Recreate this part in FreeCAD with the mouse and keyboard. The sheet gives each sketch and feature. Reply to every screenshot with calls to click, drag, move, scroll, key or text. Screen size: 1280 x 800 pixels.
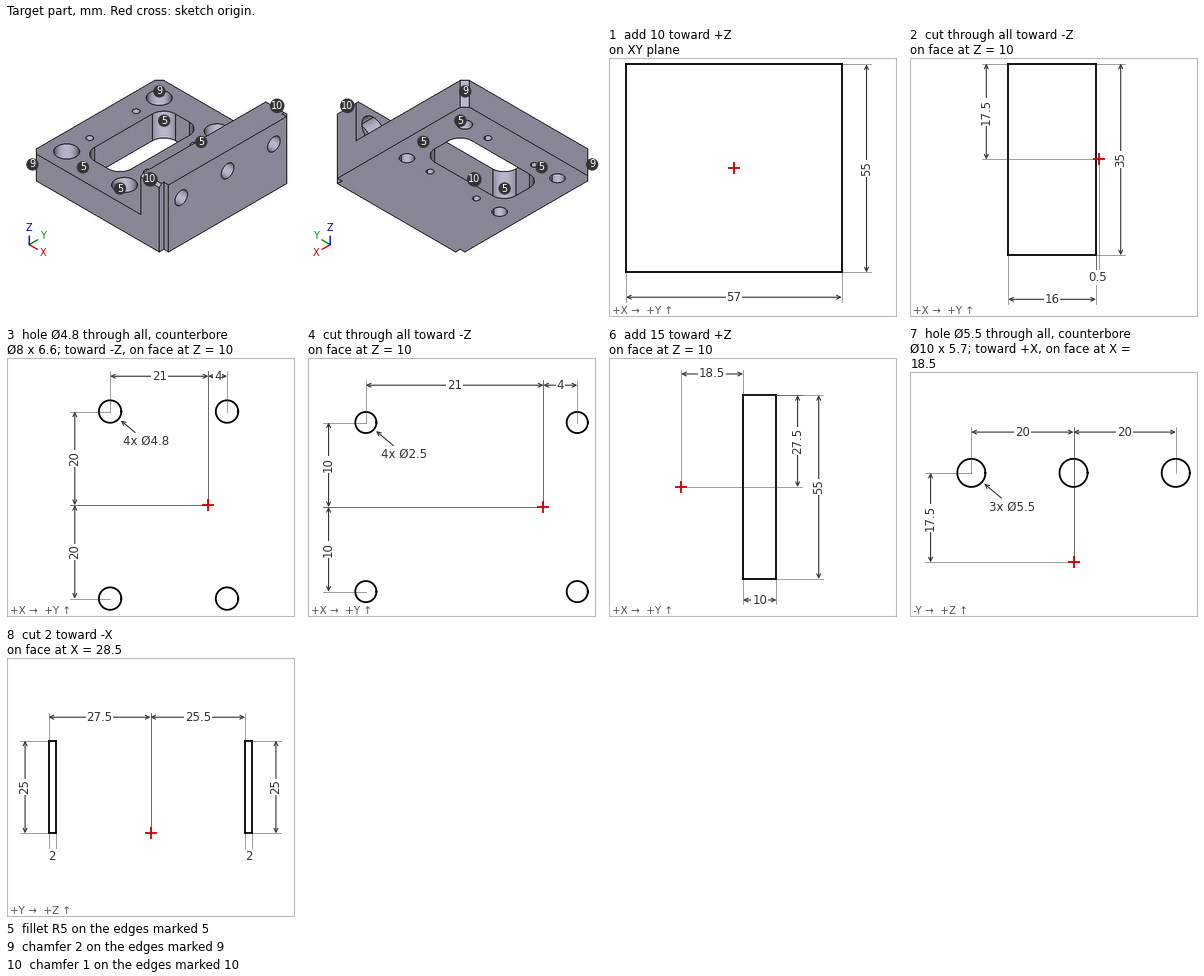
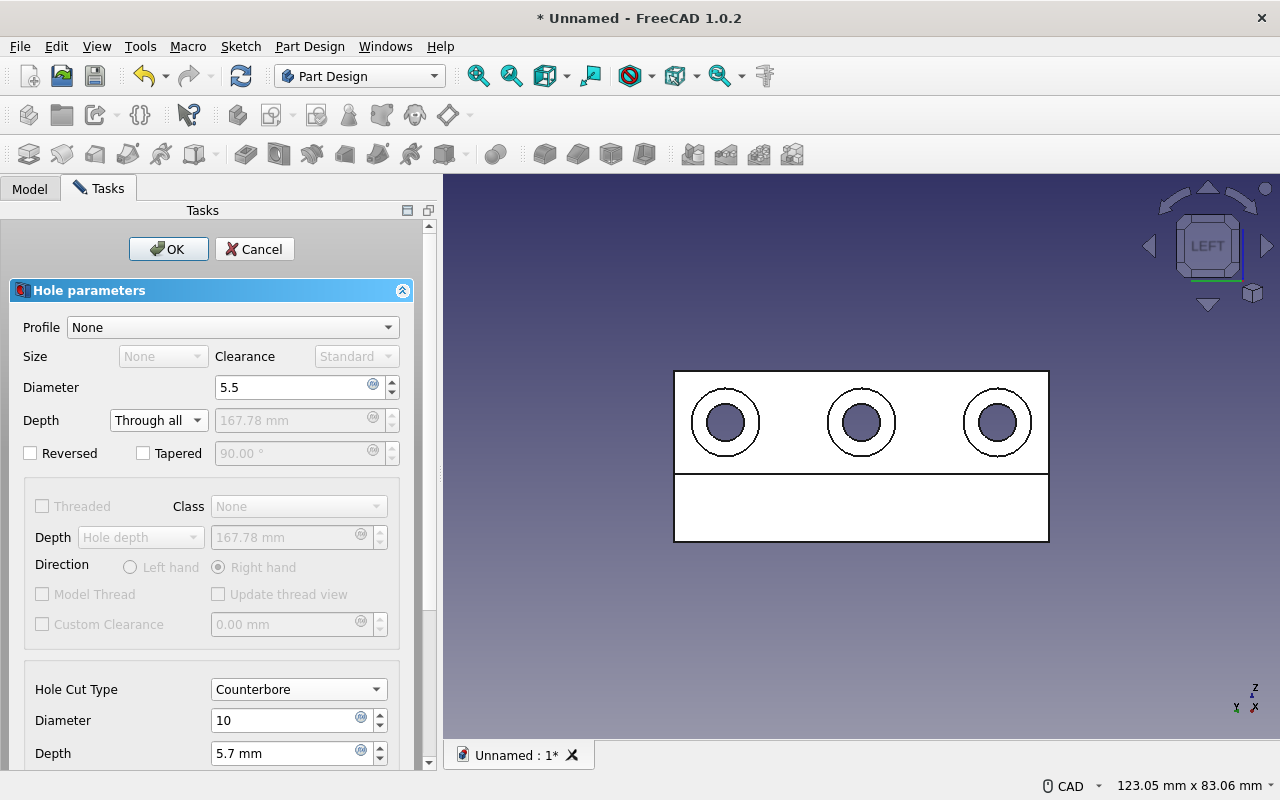
click(169, 249)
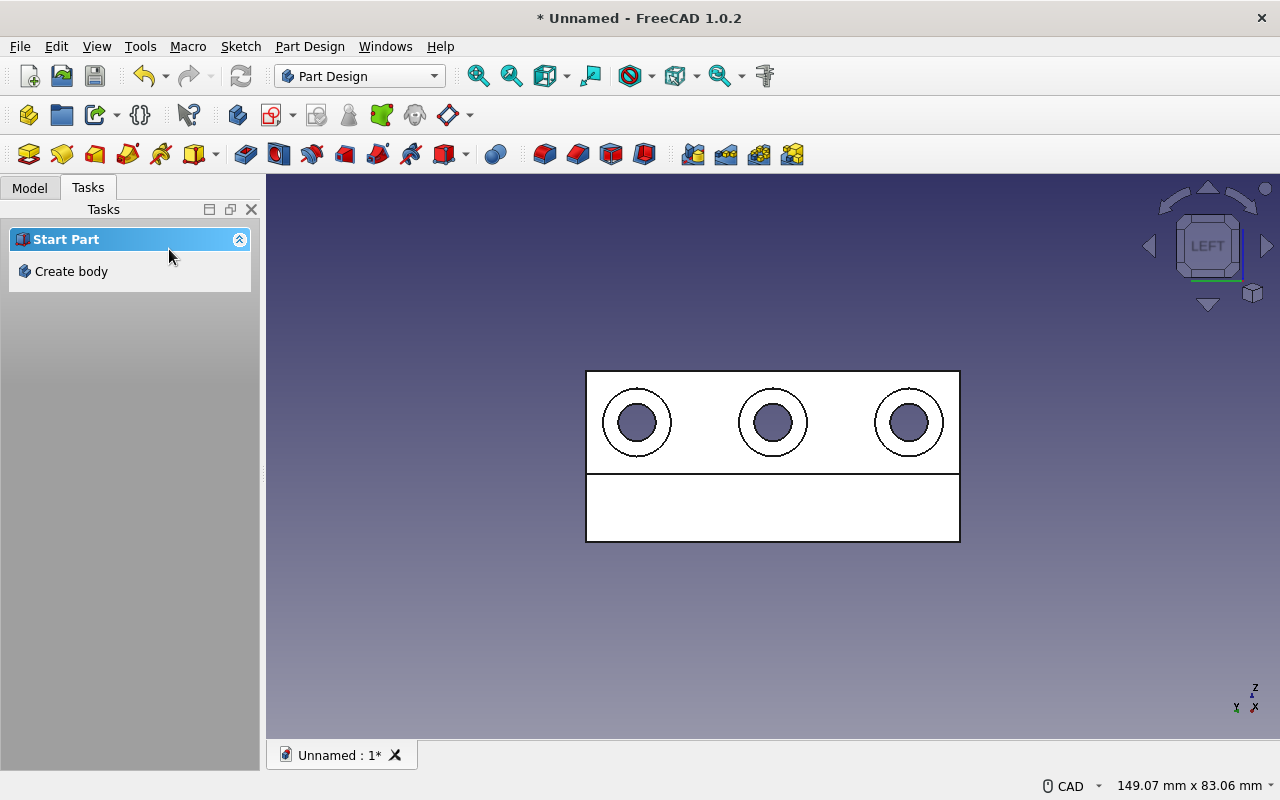
click(479, 76)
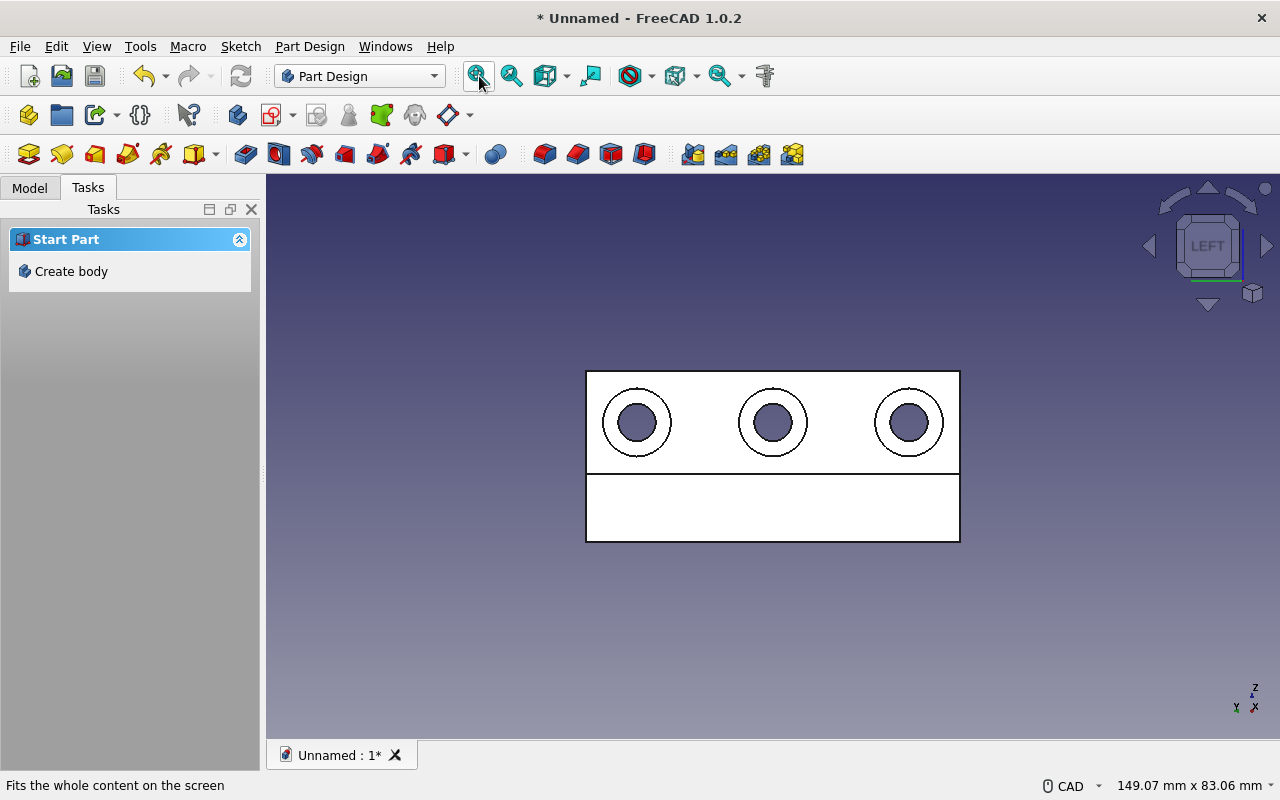
key(0)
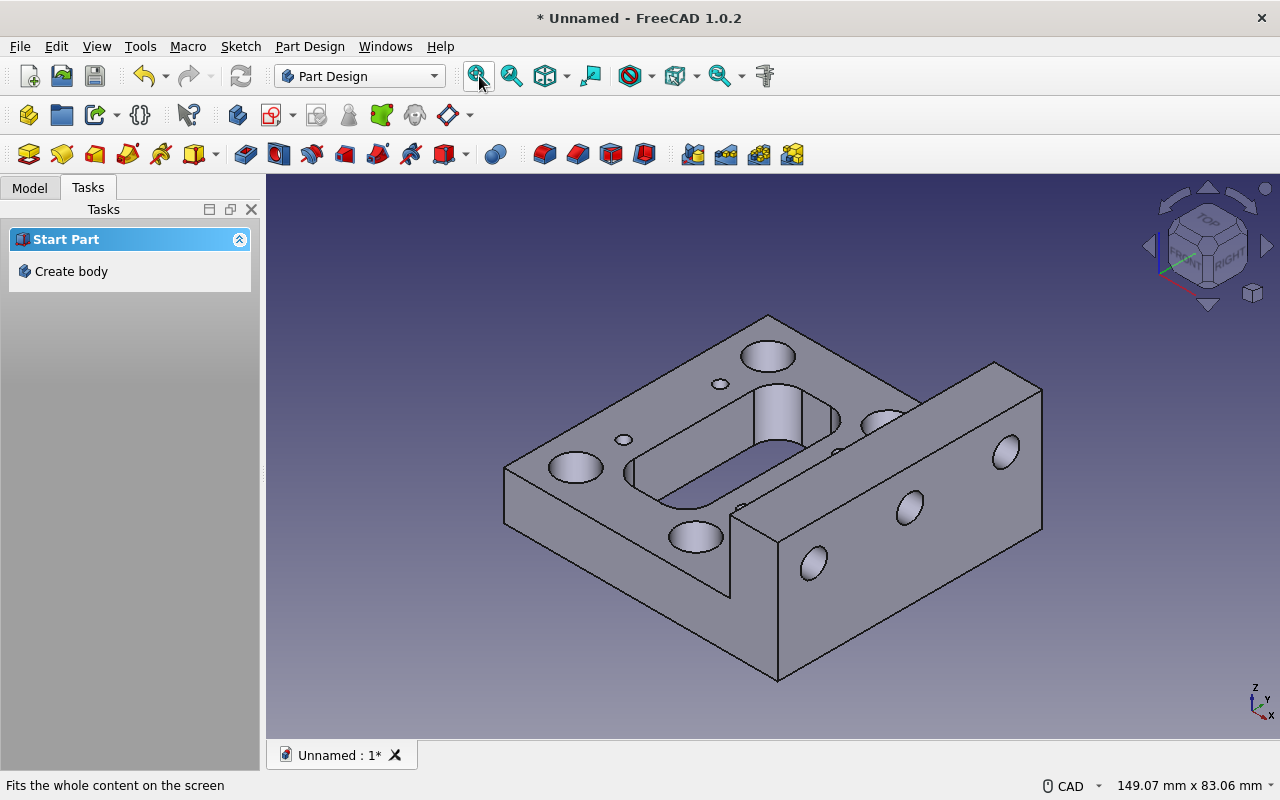
click(948, 533)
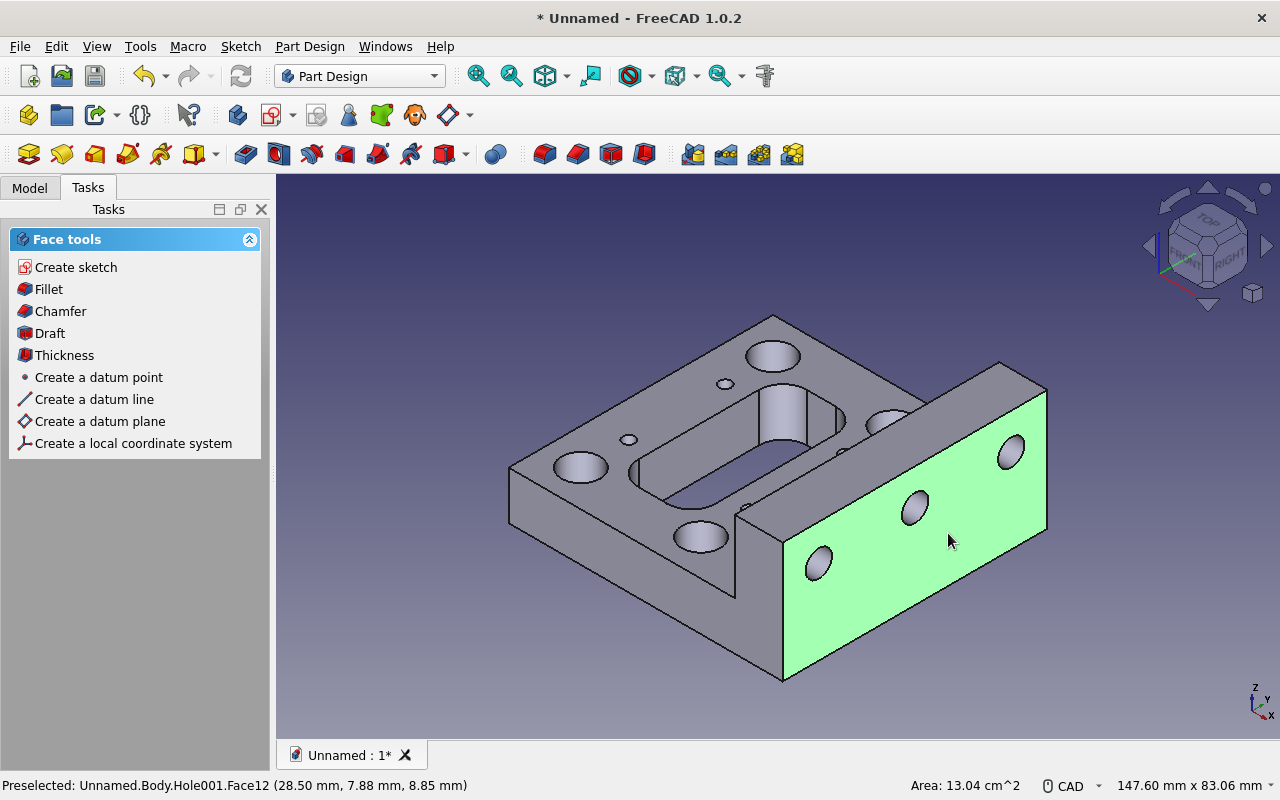
click(270, 116)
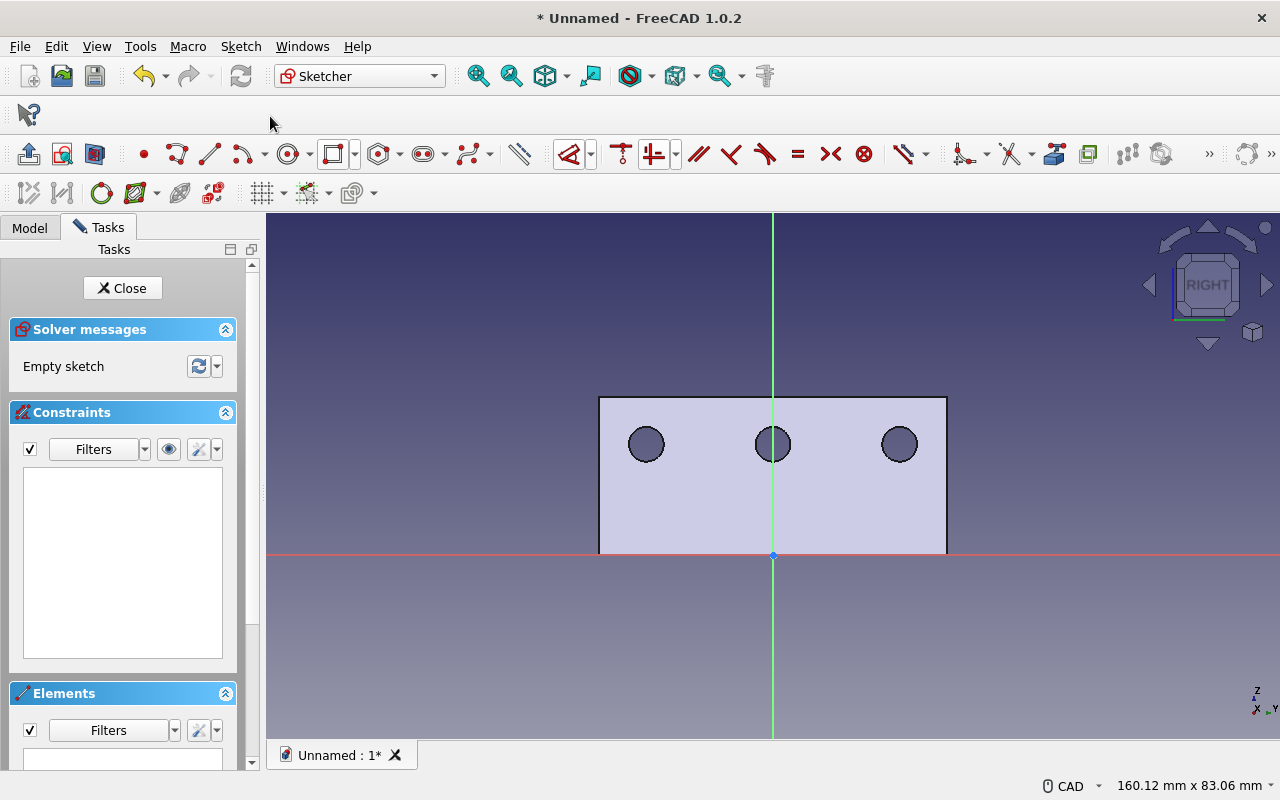
scroll(856, 476, up, 3)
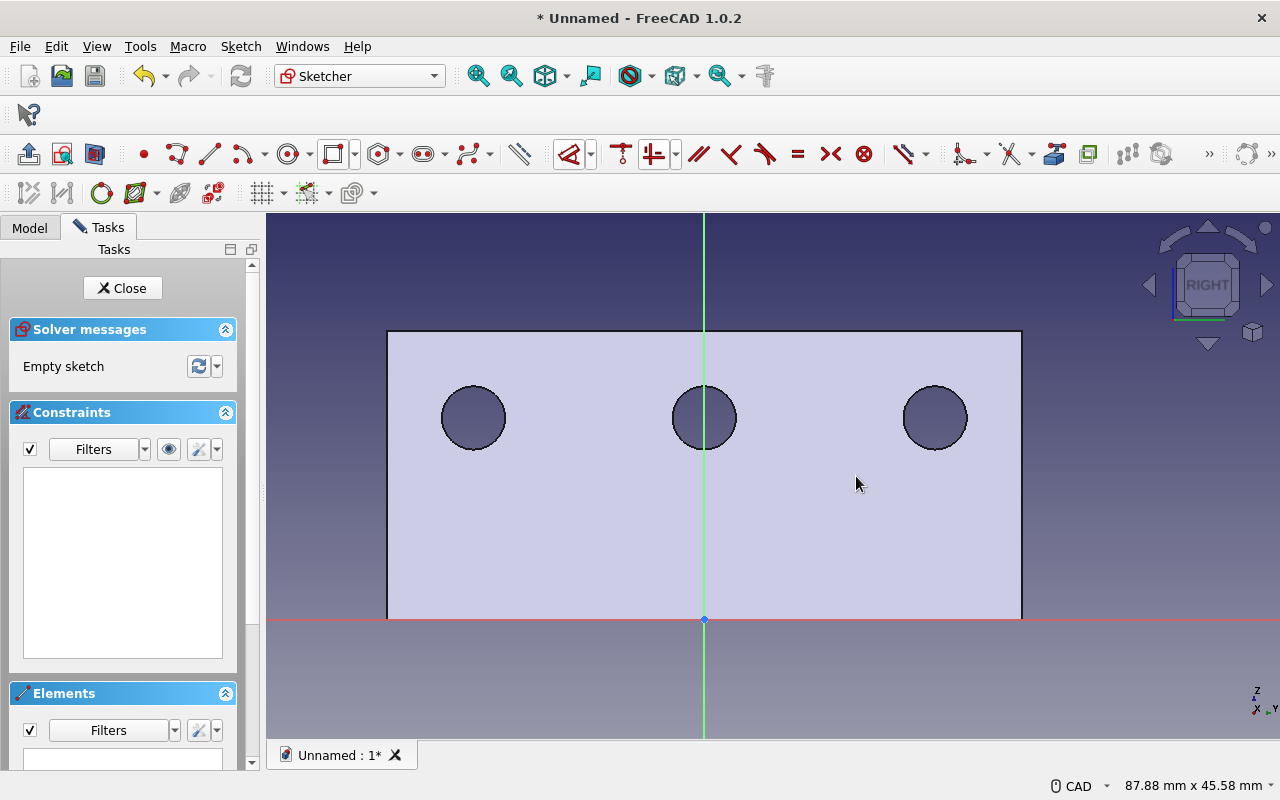
key(g)
key(r)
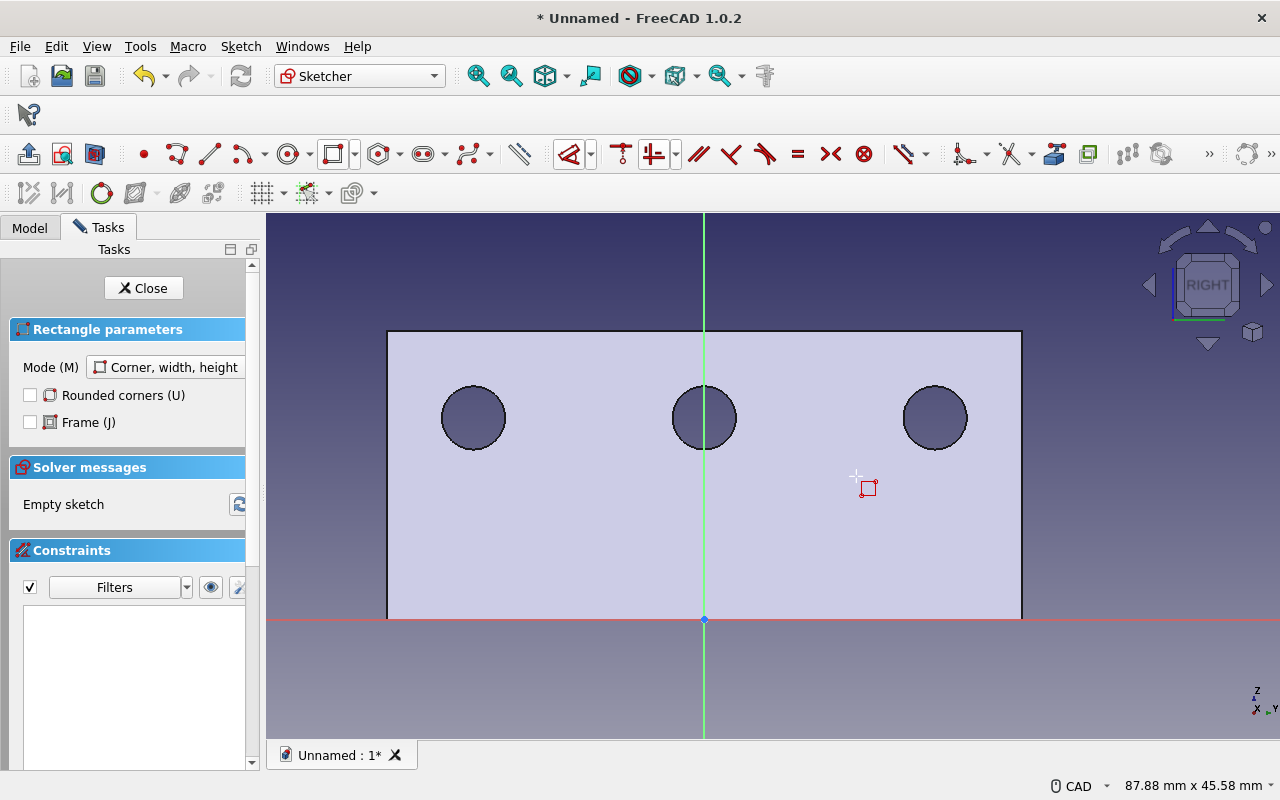
click(999, 331)
click(1022, 620)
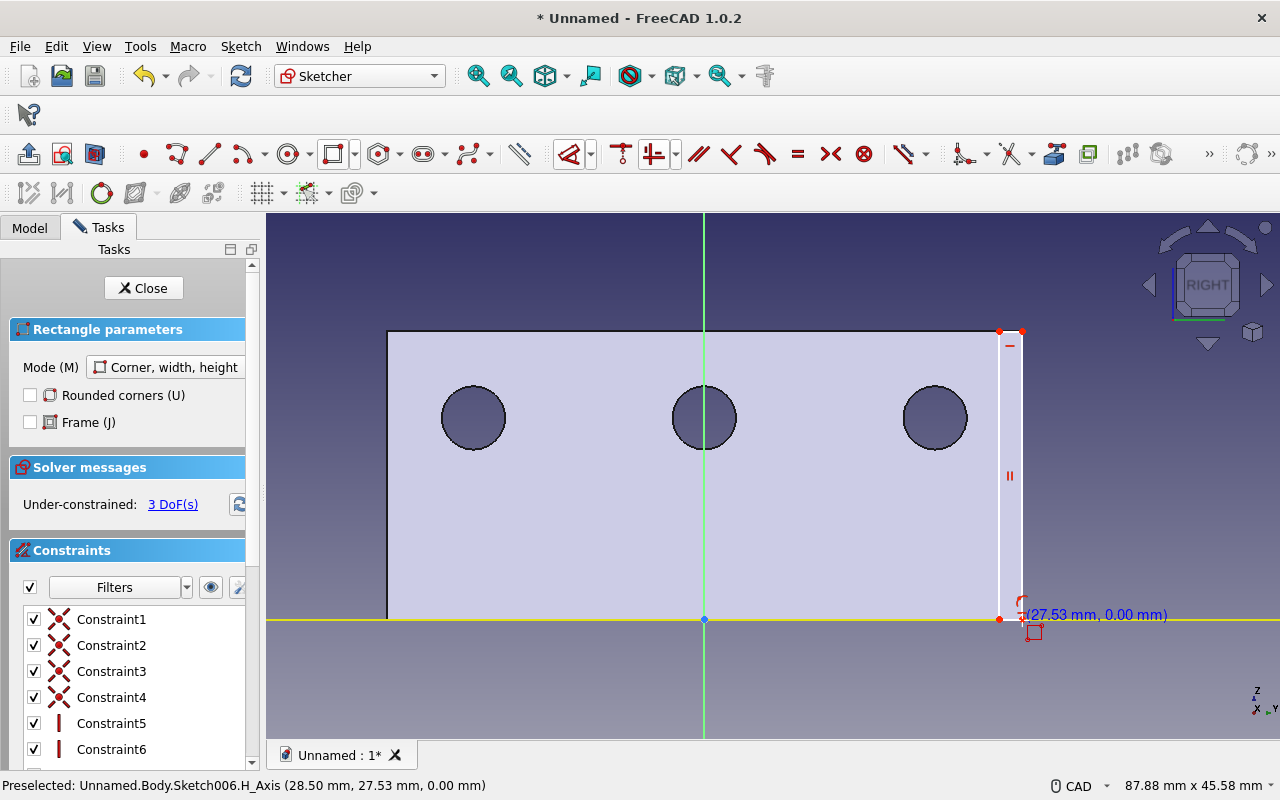
click(387, 331)
click(410, 620)
key(Escape)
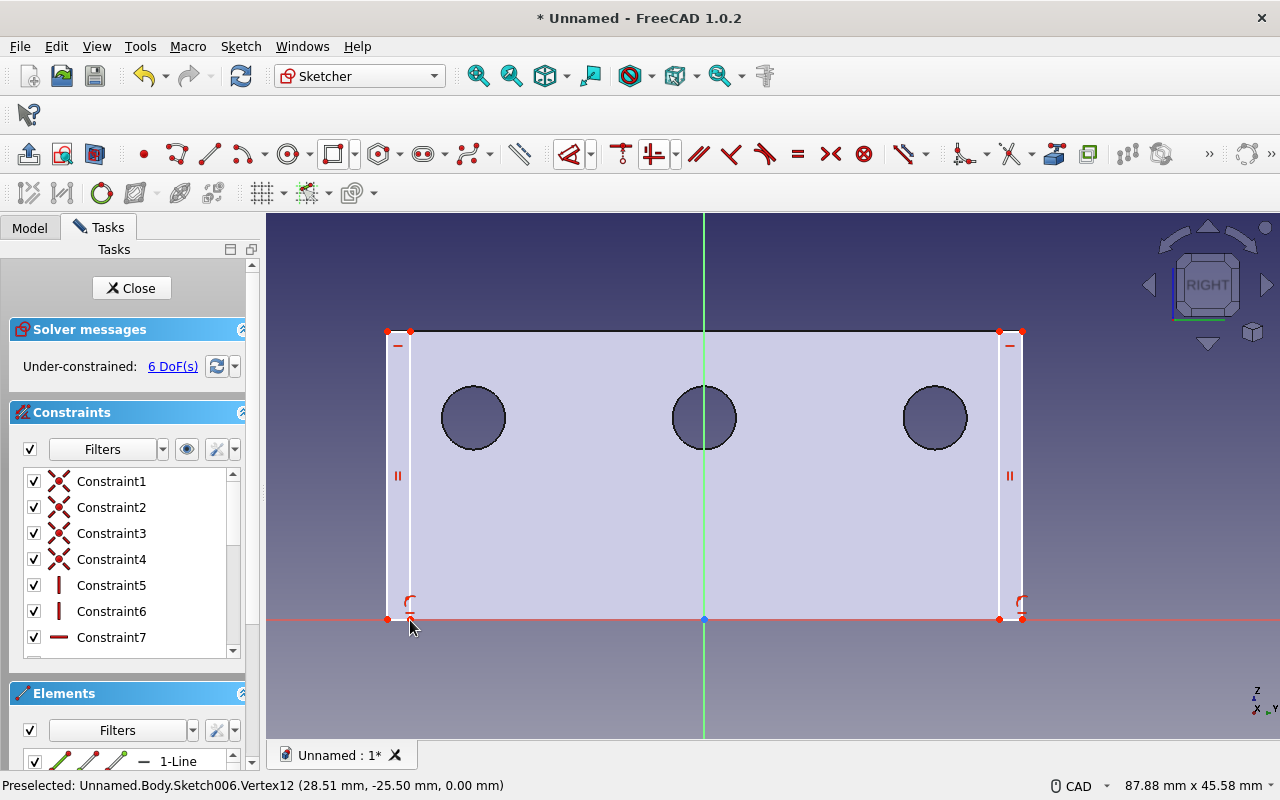
scroll(1008, 620, up, 3)